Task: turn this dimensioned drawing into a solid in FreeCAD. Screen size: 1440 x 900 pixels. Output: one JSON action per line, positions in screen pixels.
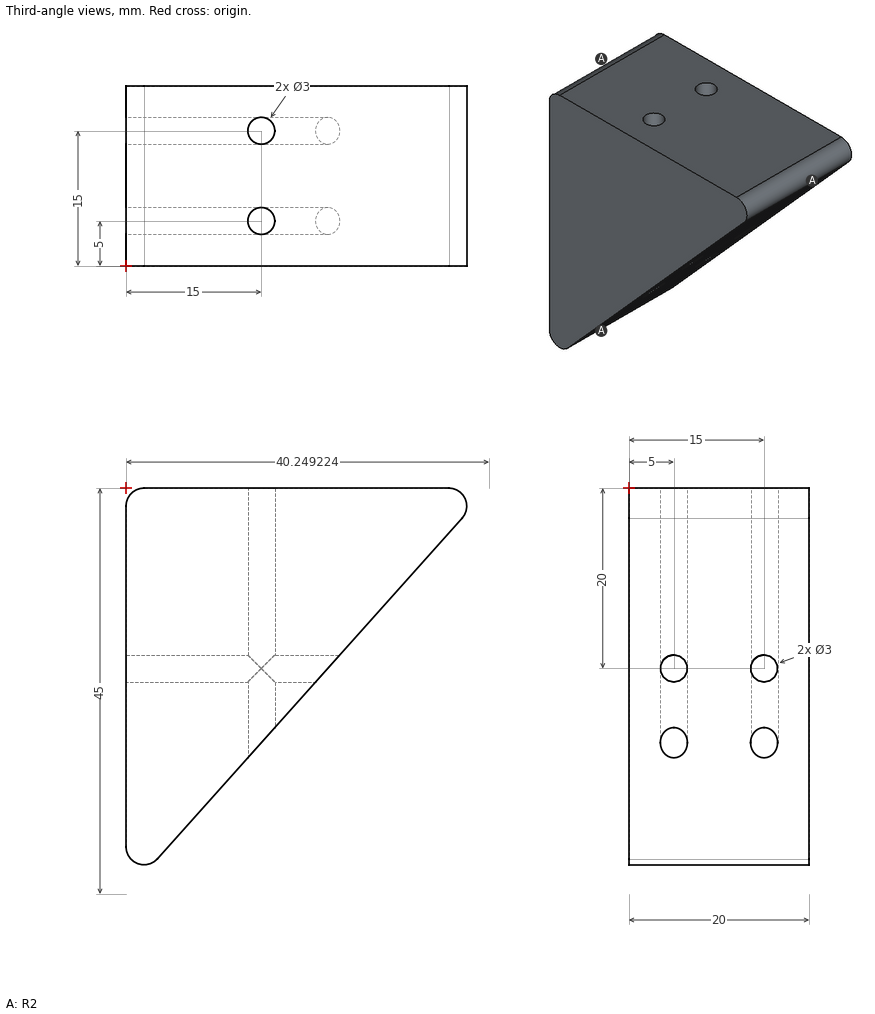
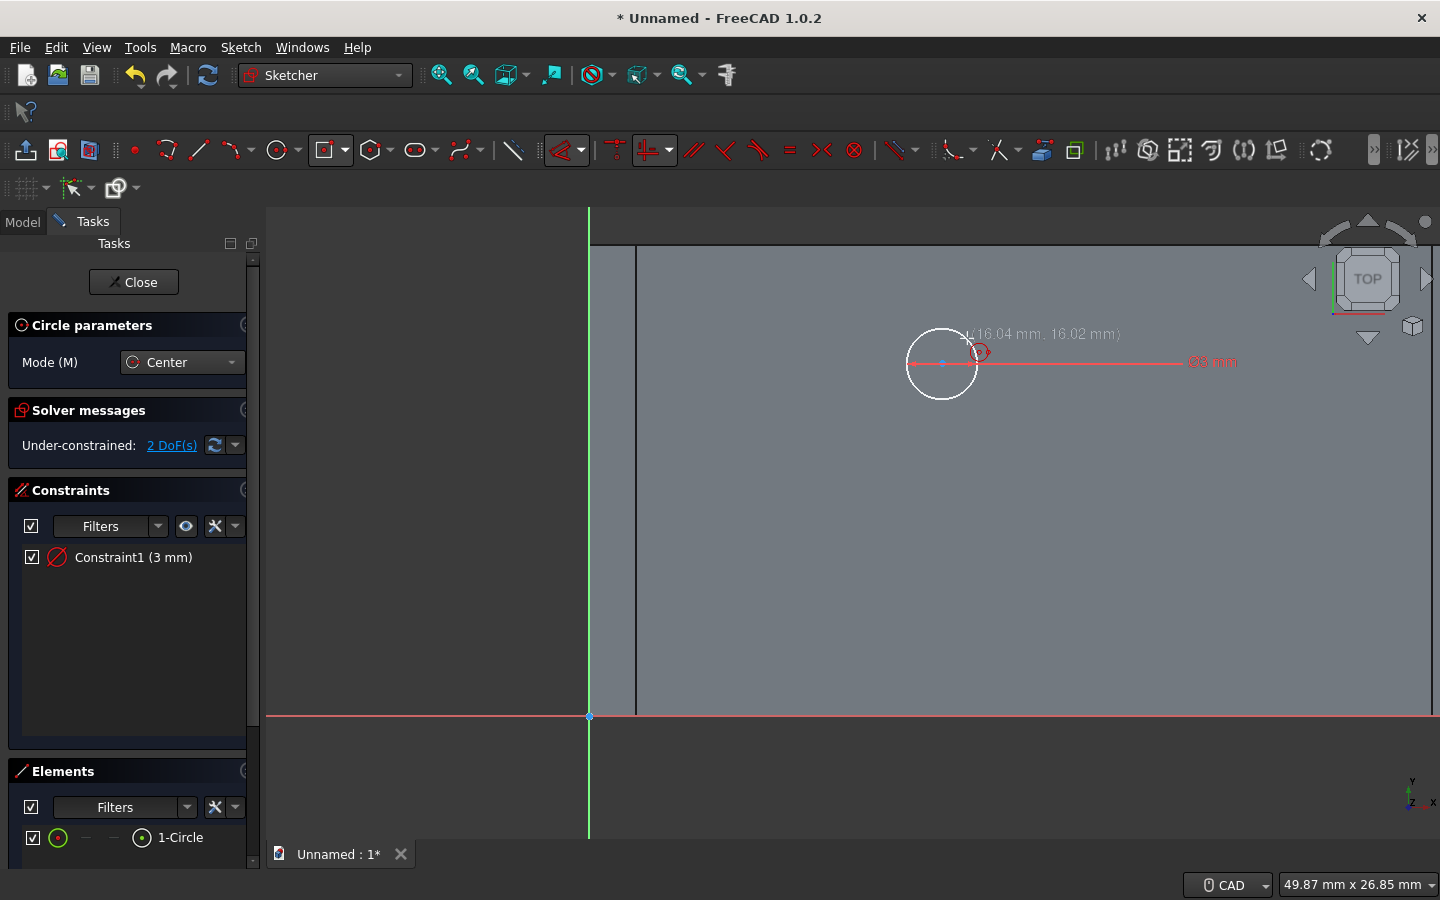
{"action": "left_click", "coordinate": [942, 598]}
{"action": "mouse_move", "coordinate": [967, 573]}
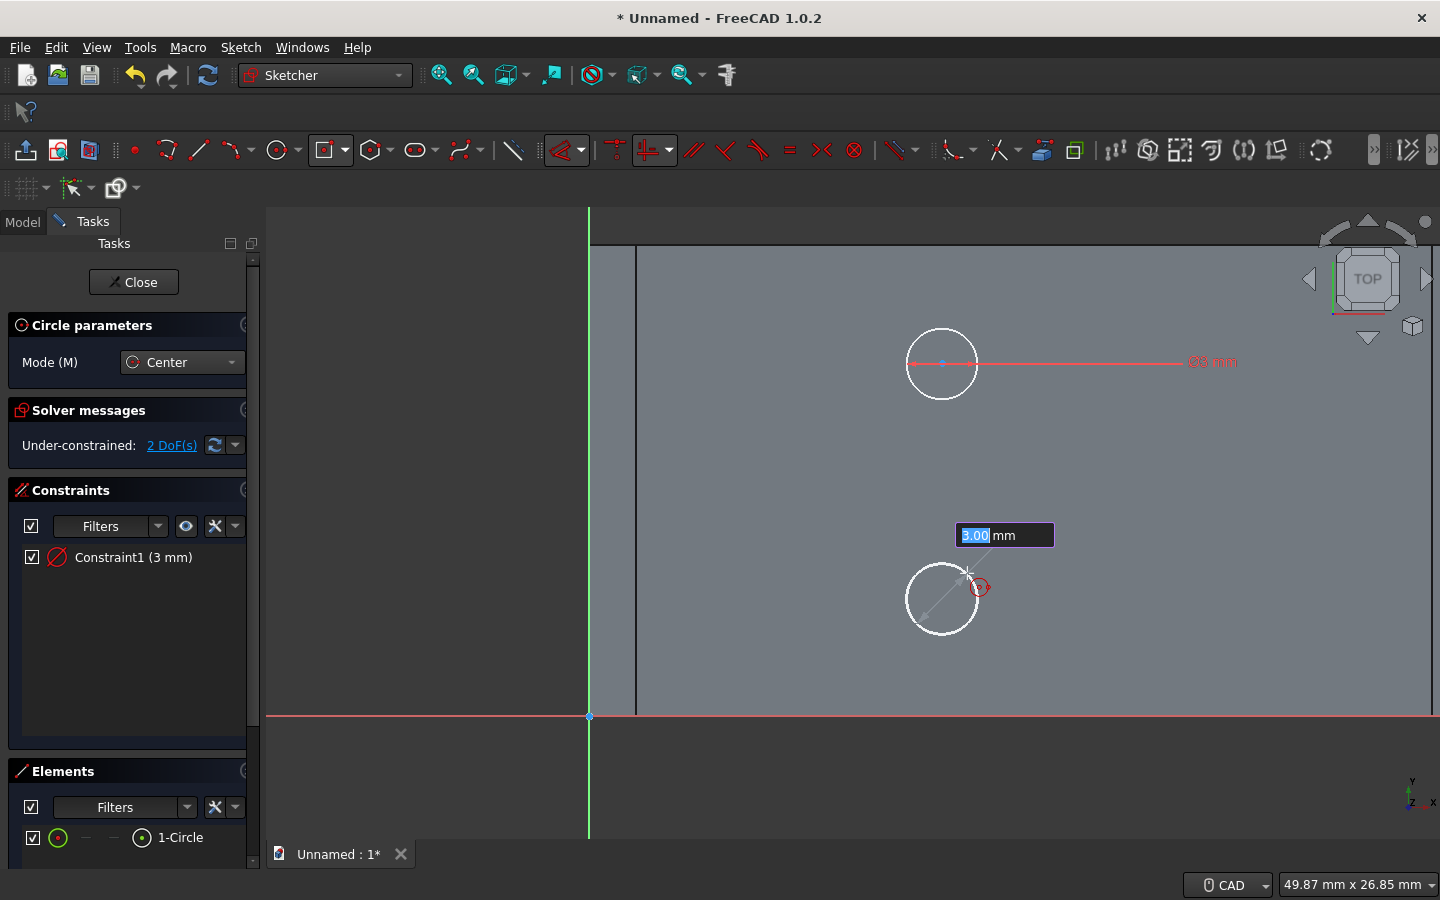
{"action": "type", "text": "3"}
{"action": "key", "text": "Return"}
{"action": "key", "text": "Escape"}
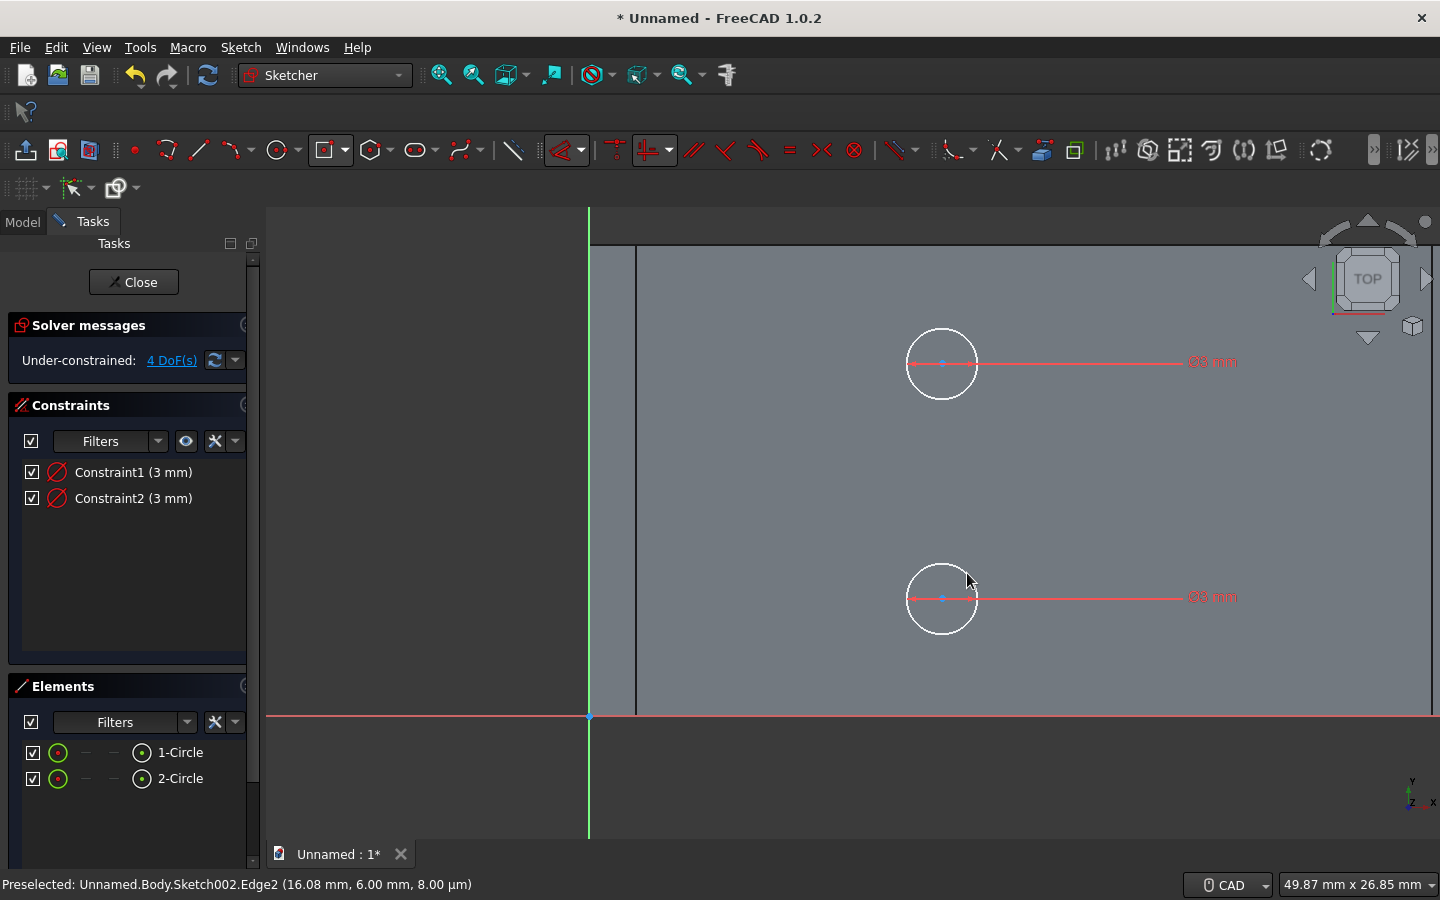
{"action": "left_click", "coordinate": [942, 364]}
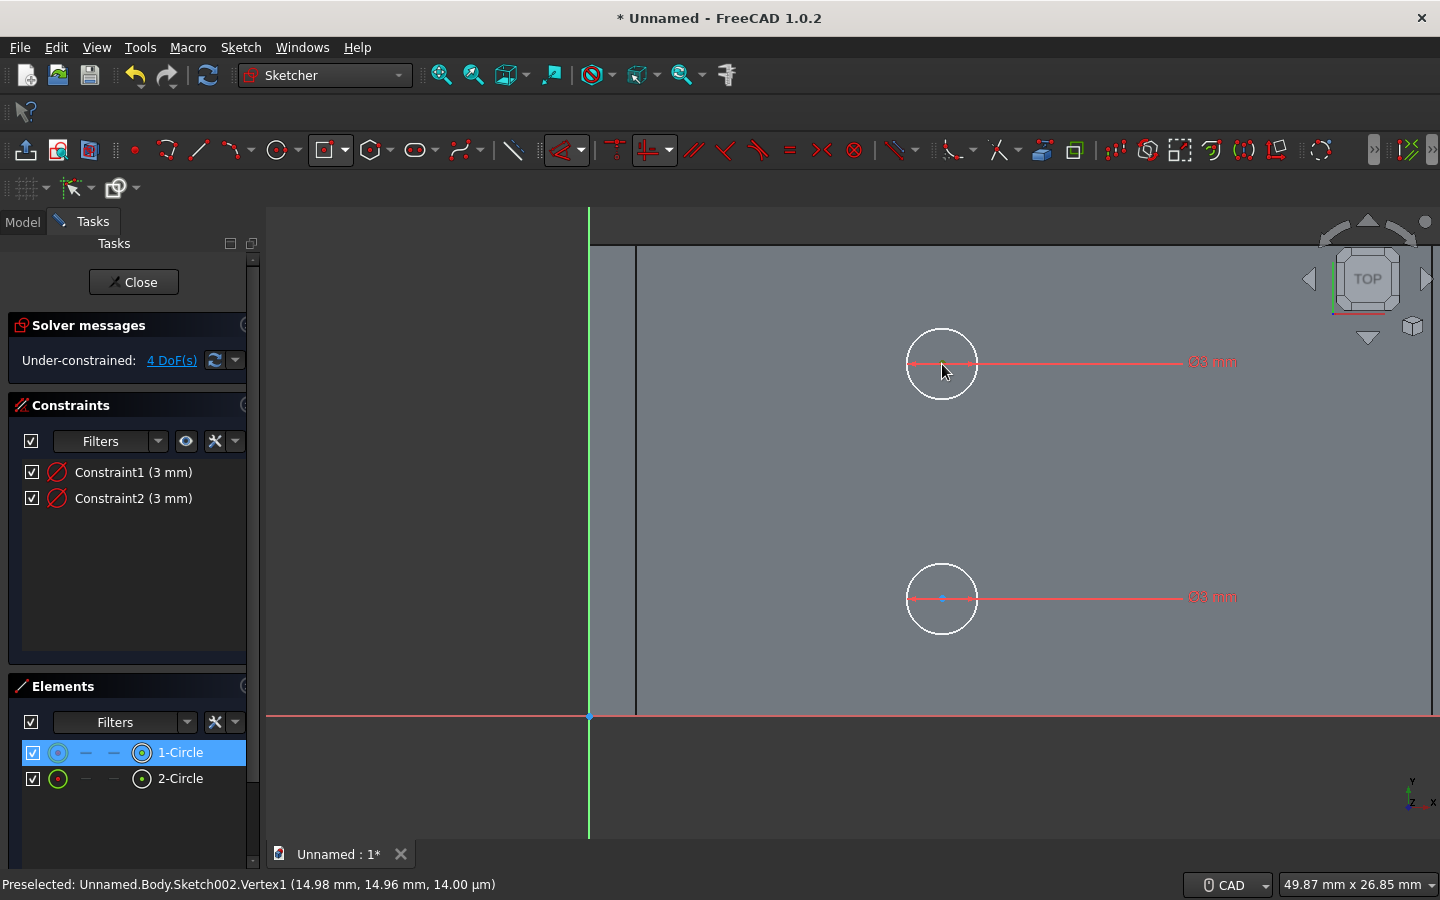
{"action": "left_click", "coordinate": [942, 599]}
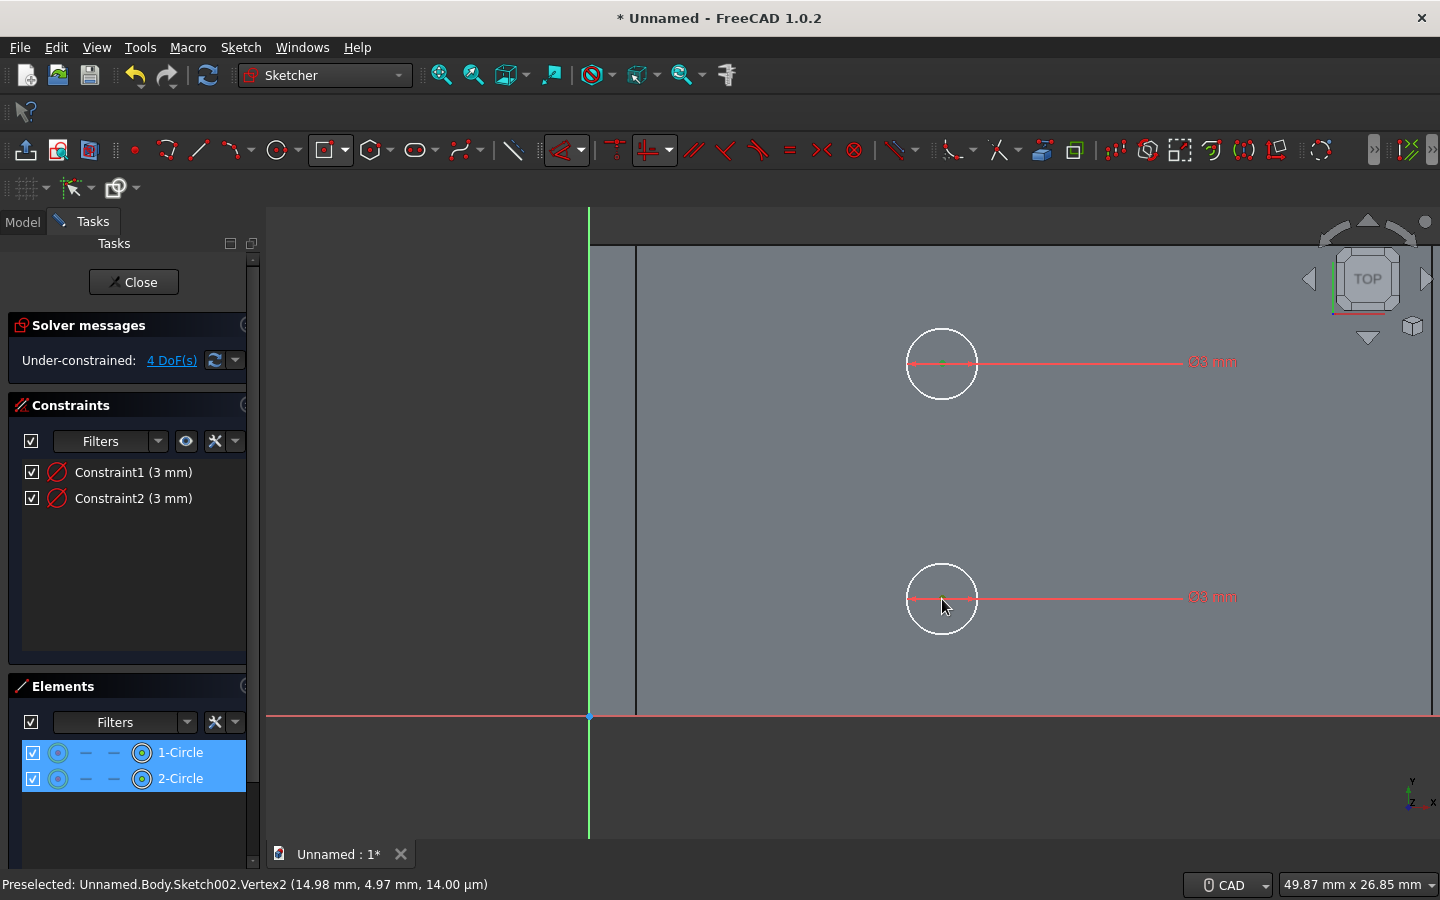
{"action": "key", "text": "v"}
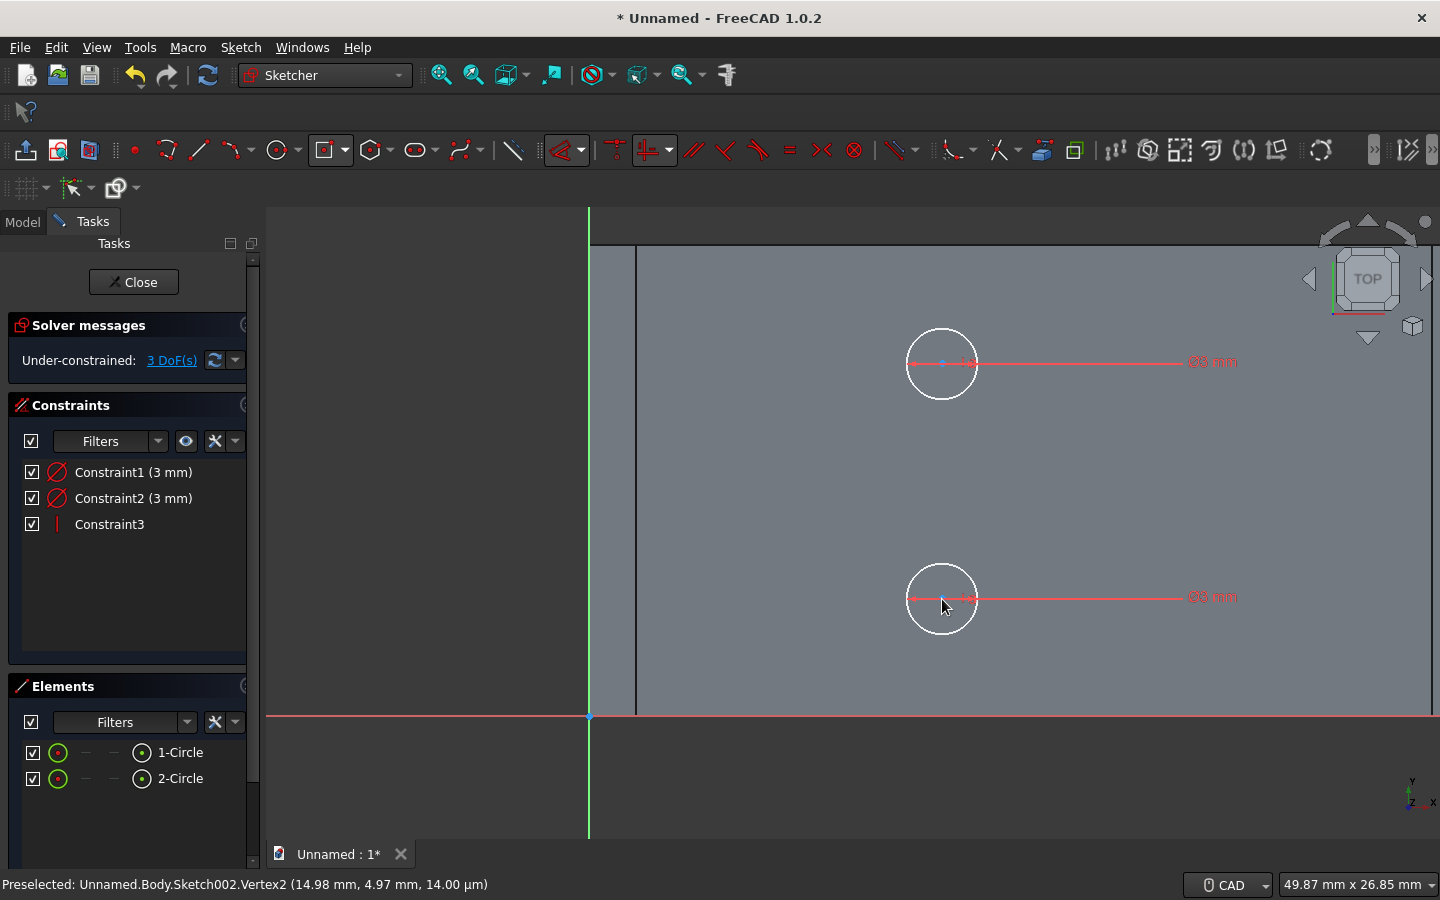
{"action": "left_click", "coordinate": [560, 150]}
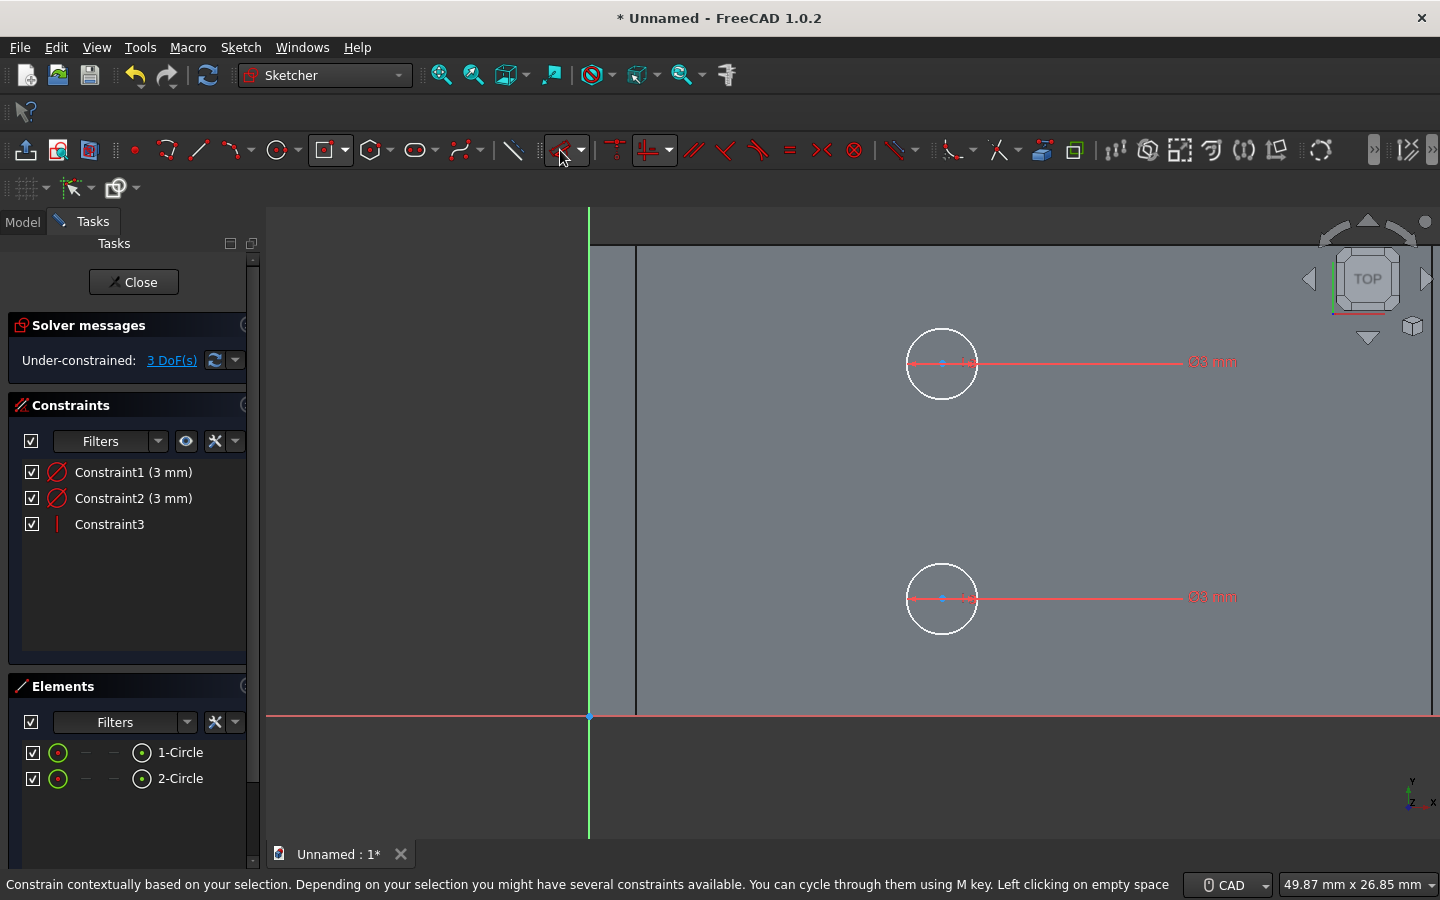
{"action": "left_click", "coordinate": [942, 599]}
{"action": "left_click", "coordinate": [555, 658]}